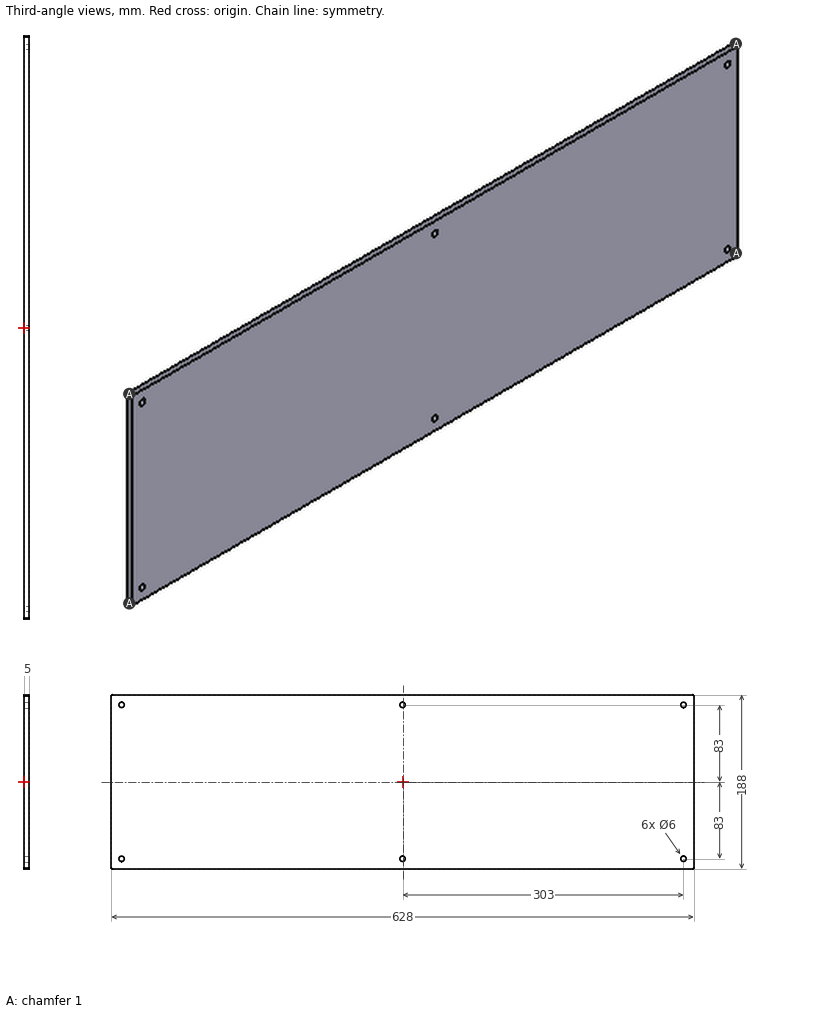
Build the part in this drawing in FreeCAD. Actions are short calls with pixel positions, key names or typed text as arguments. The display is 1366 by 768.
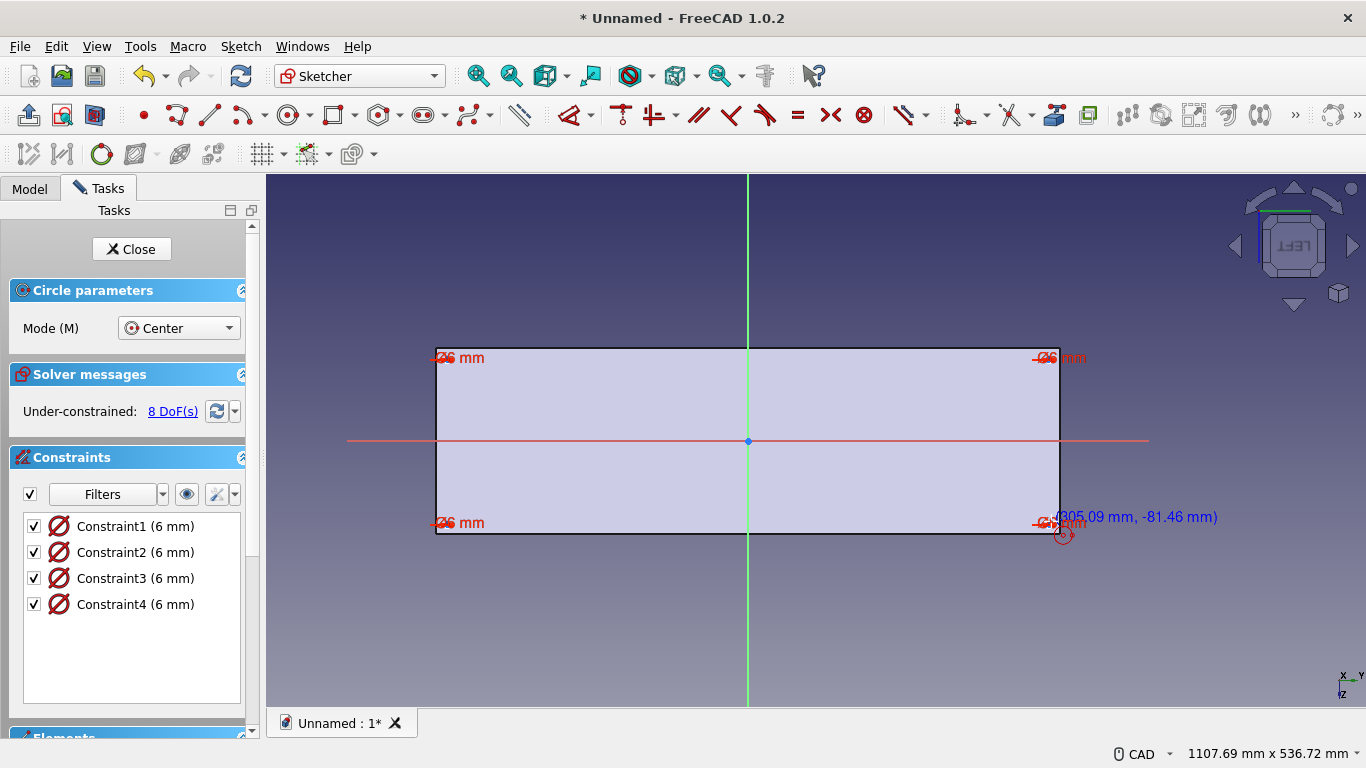
scroll(748, 524, up, 11)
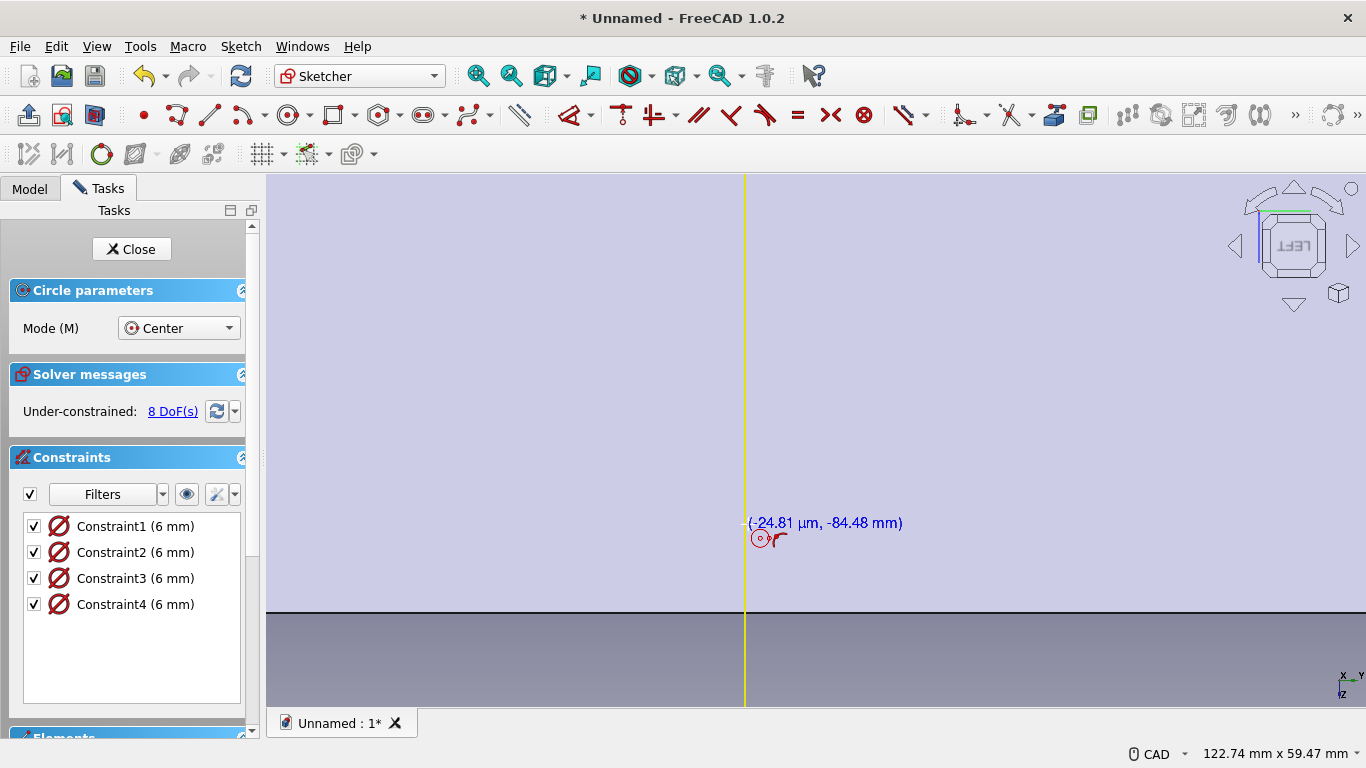
scroll(748, 524, down, 11)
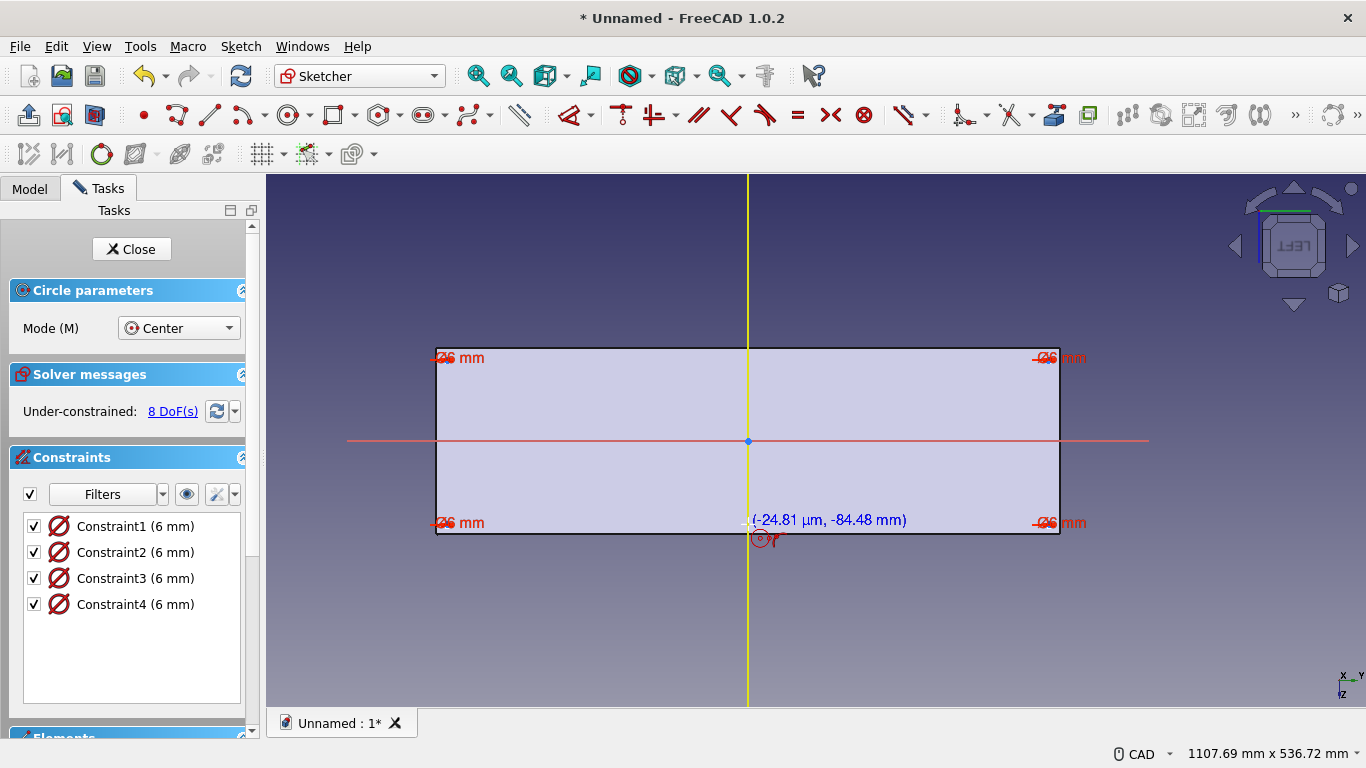
click(748, 524)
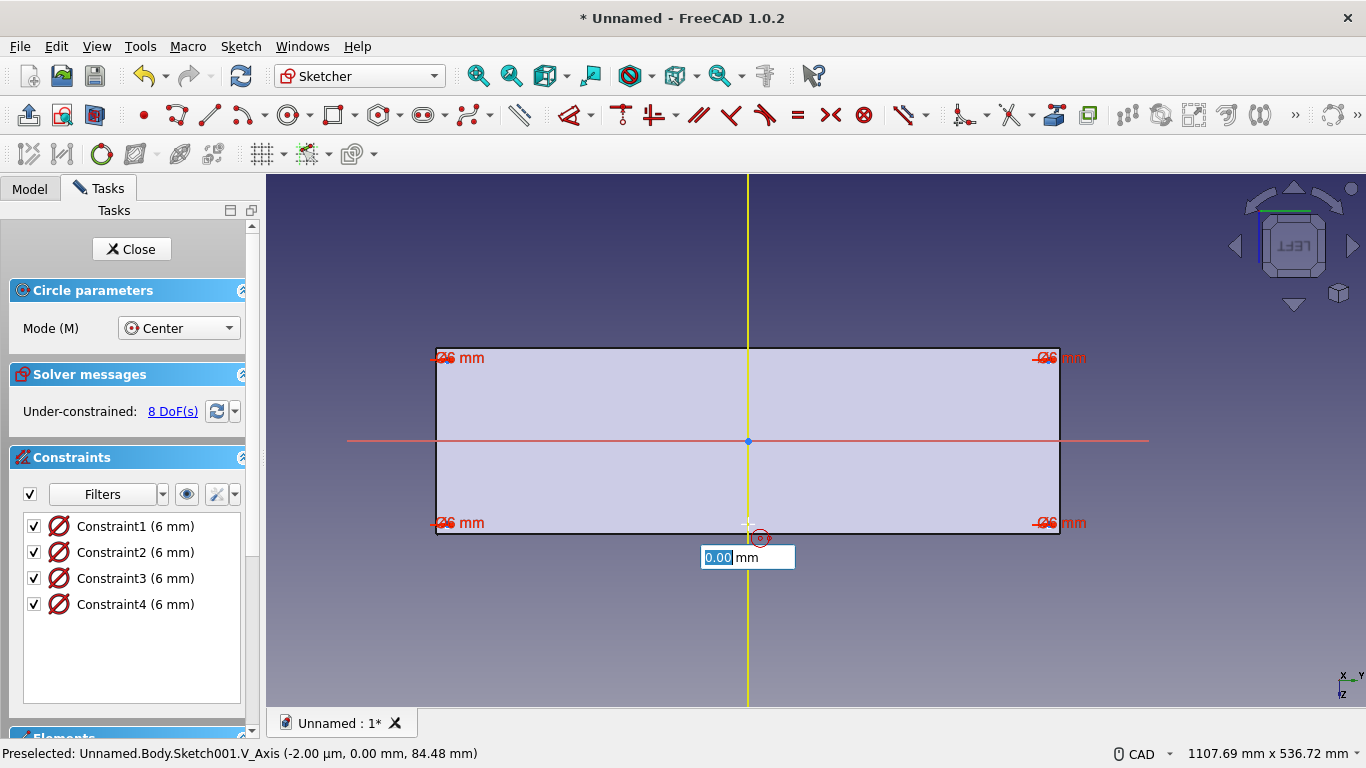
scroll(751, 523, up, 9)
move(748, 517)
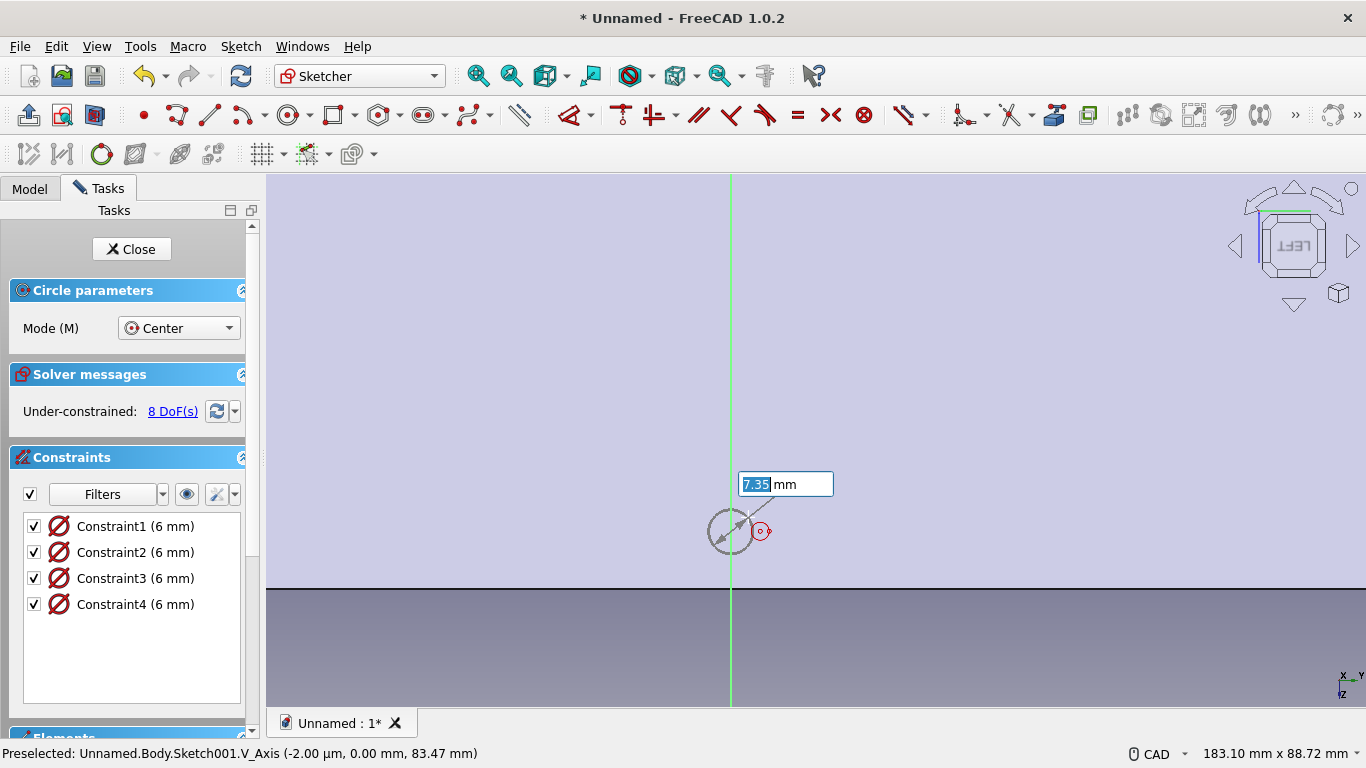
text(6)
key(Return)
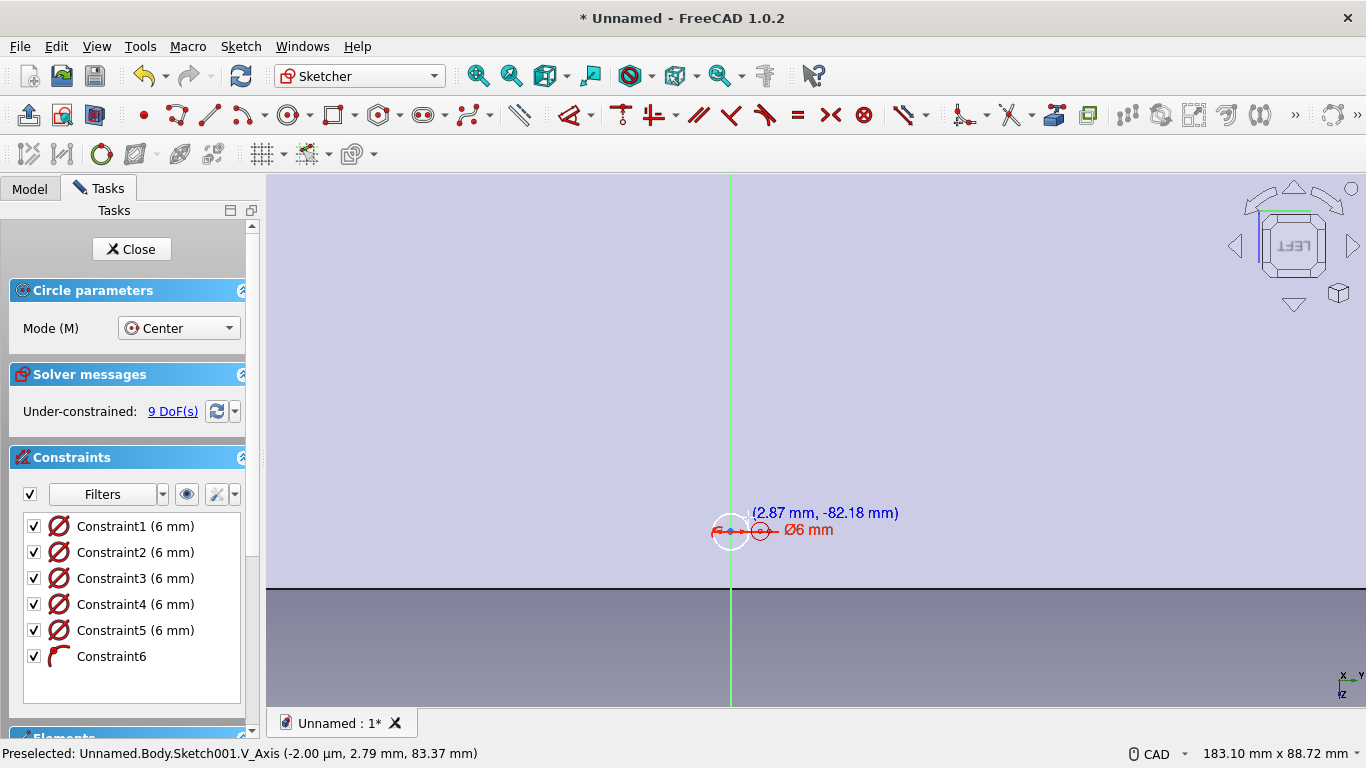
scroll(751, 523, down, 9)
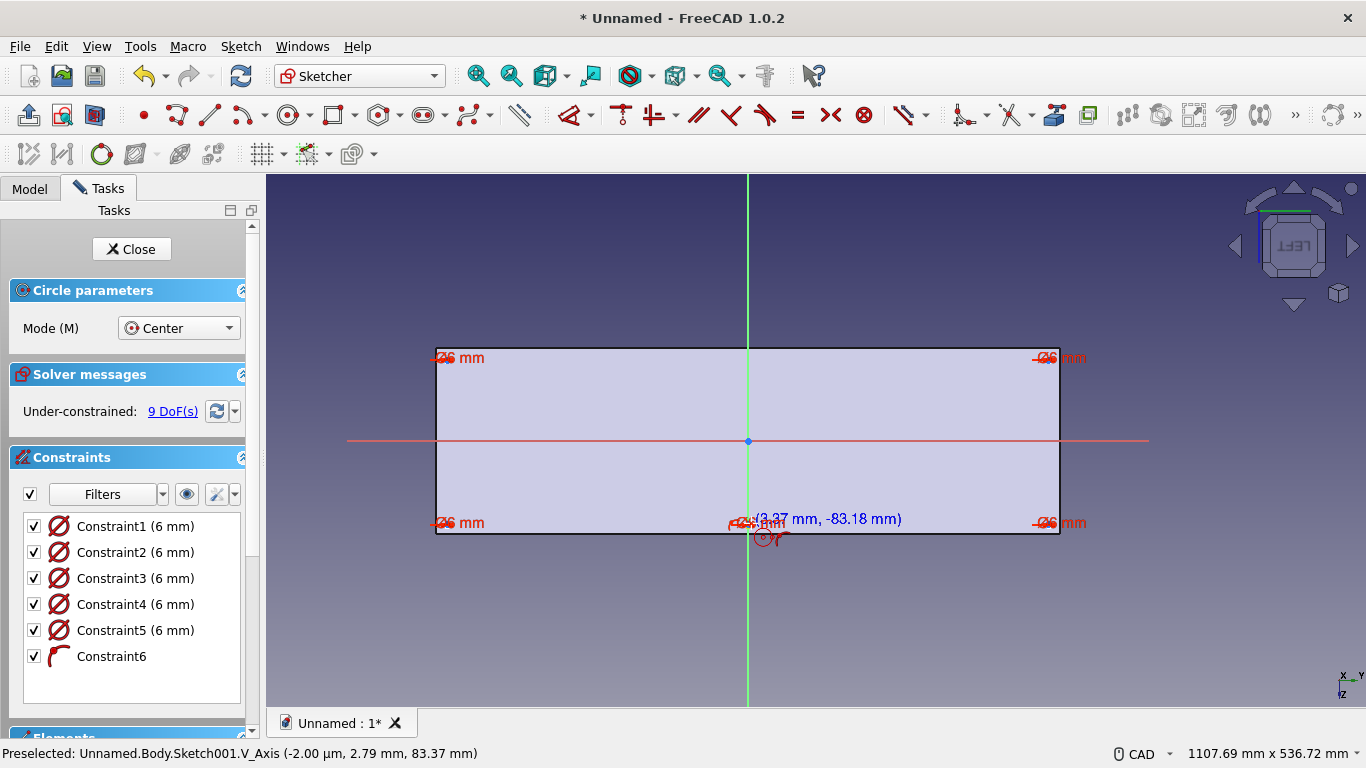
scroll(748, 359, up, 11)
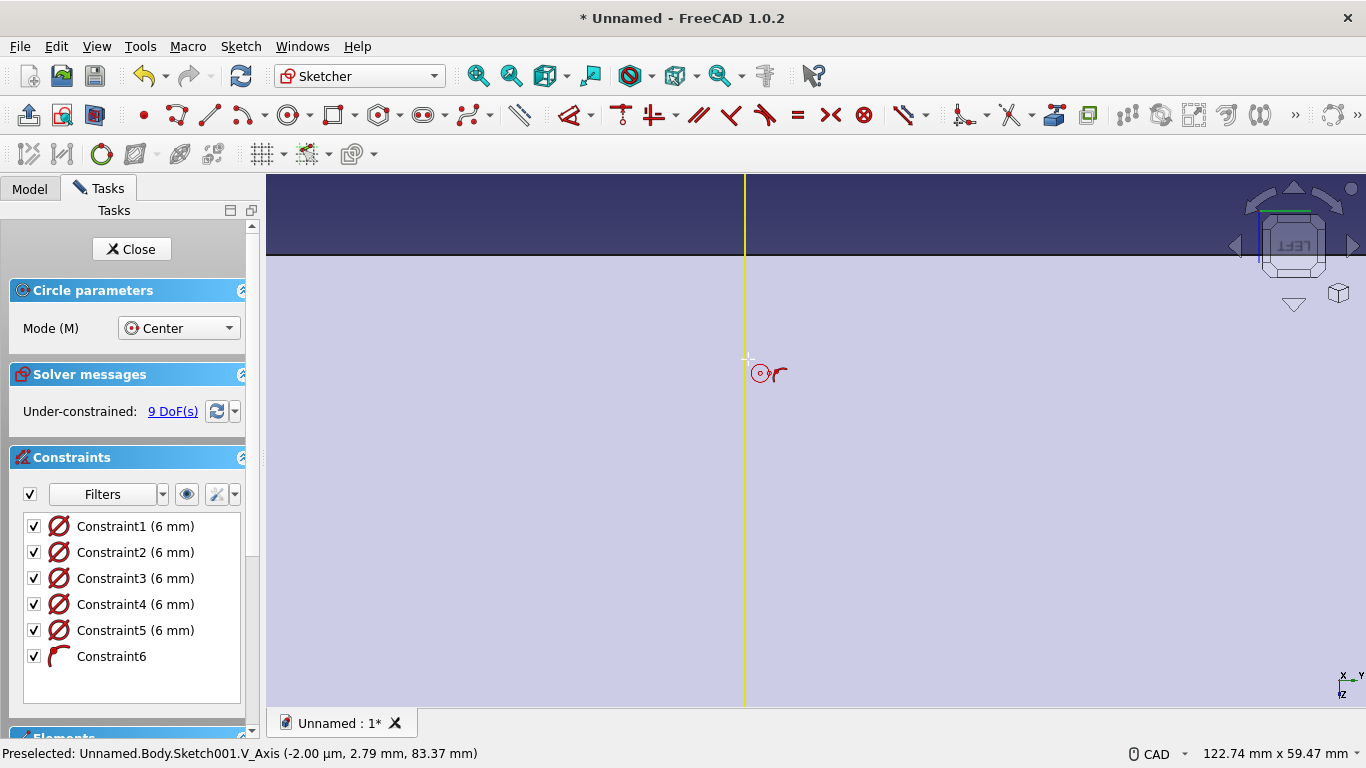
scroll(748, 359, down, 11)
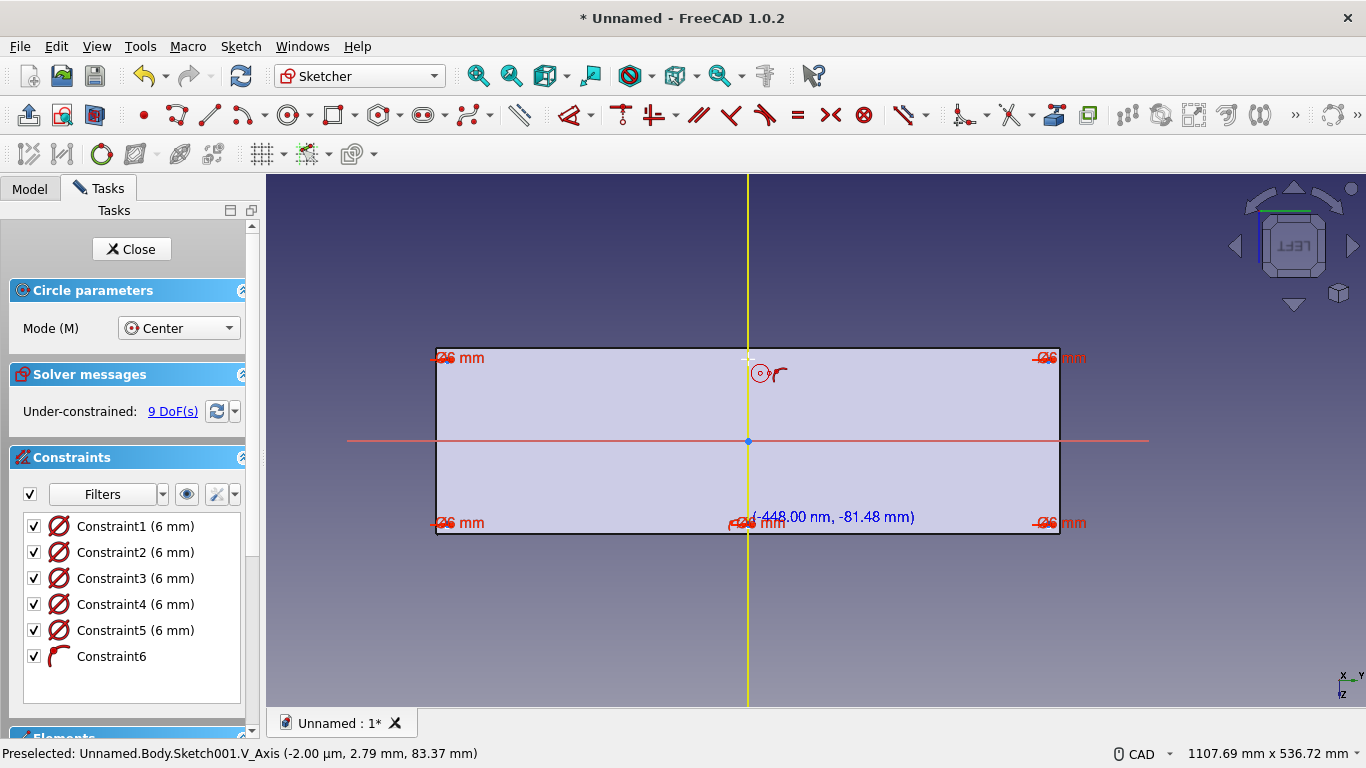
click(748, 359)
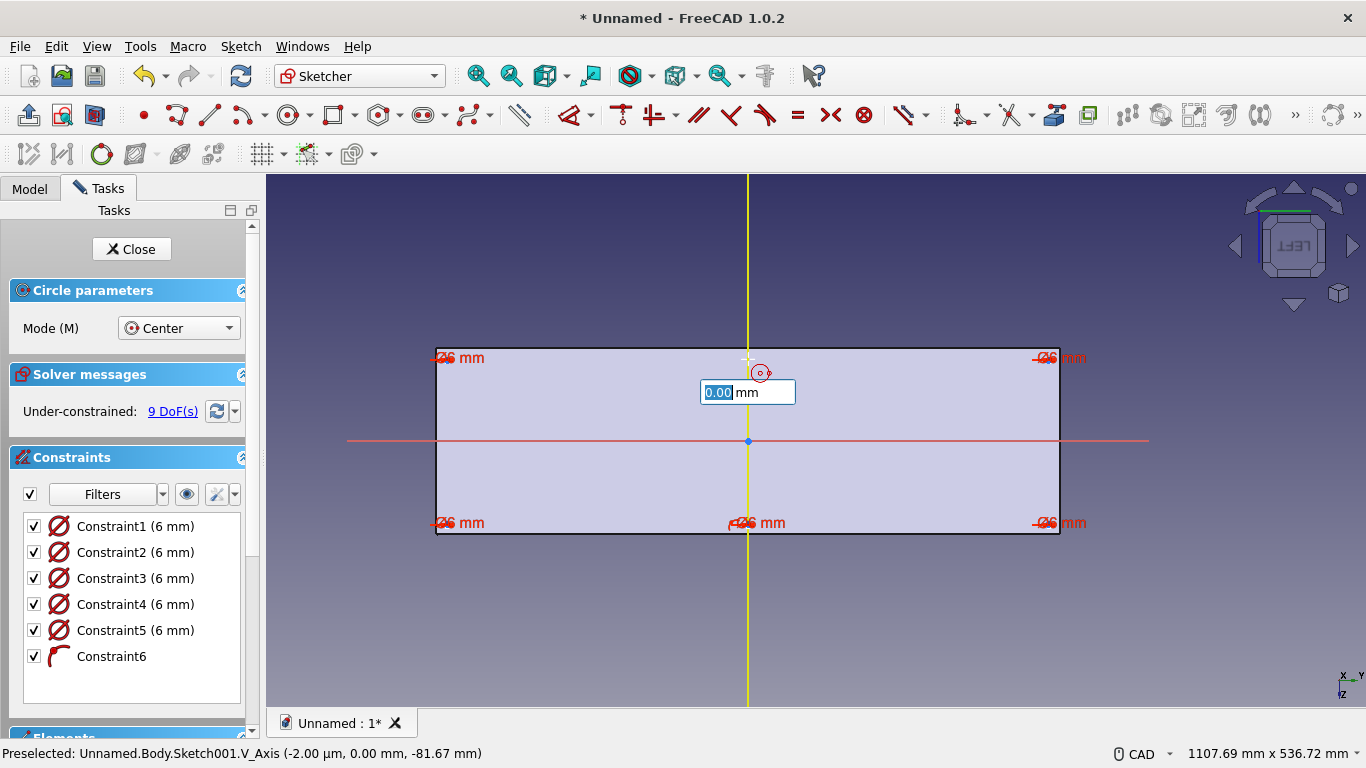
scroll(751, 358, up, 9)
move(748, 354)